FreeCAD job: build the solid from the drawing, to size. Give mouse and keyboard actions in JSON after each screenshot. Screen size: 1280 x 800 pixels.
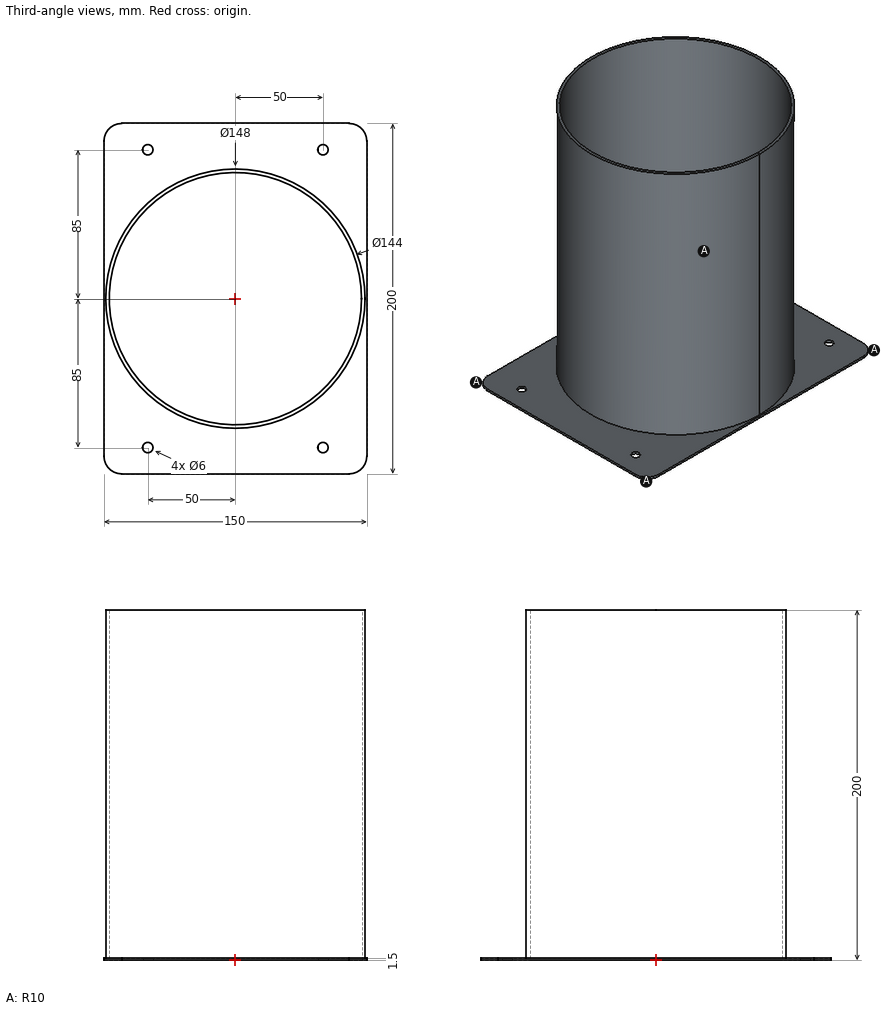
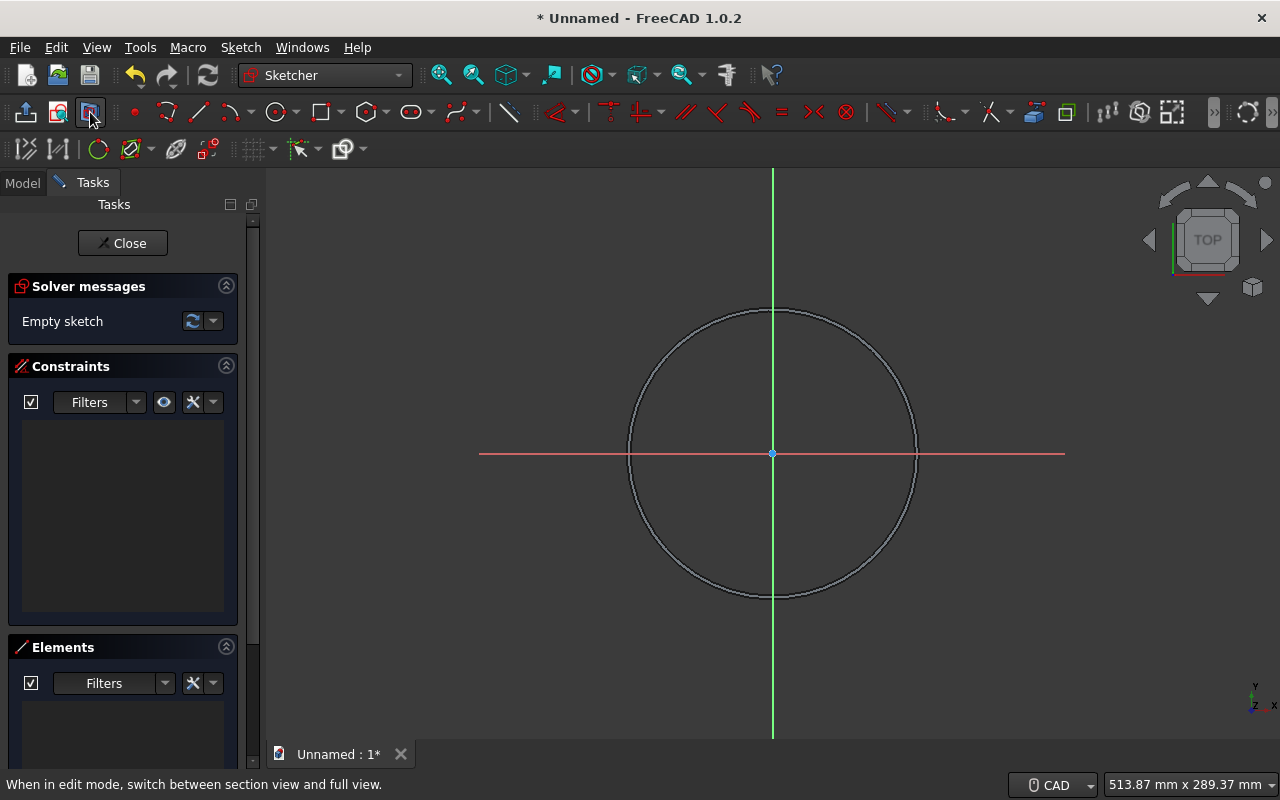
{"action": "left_click", "coordinate": [344, 112]}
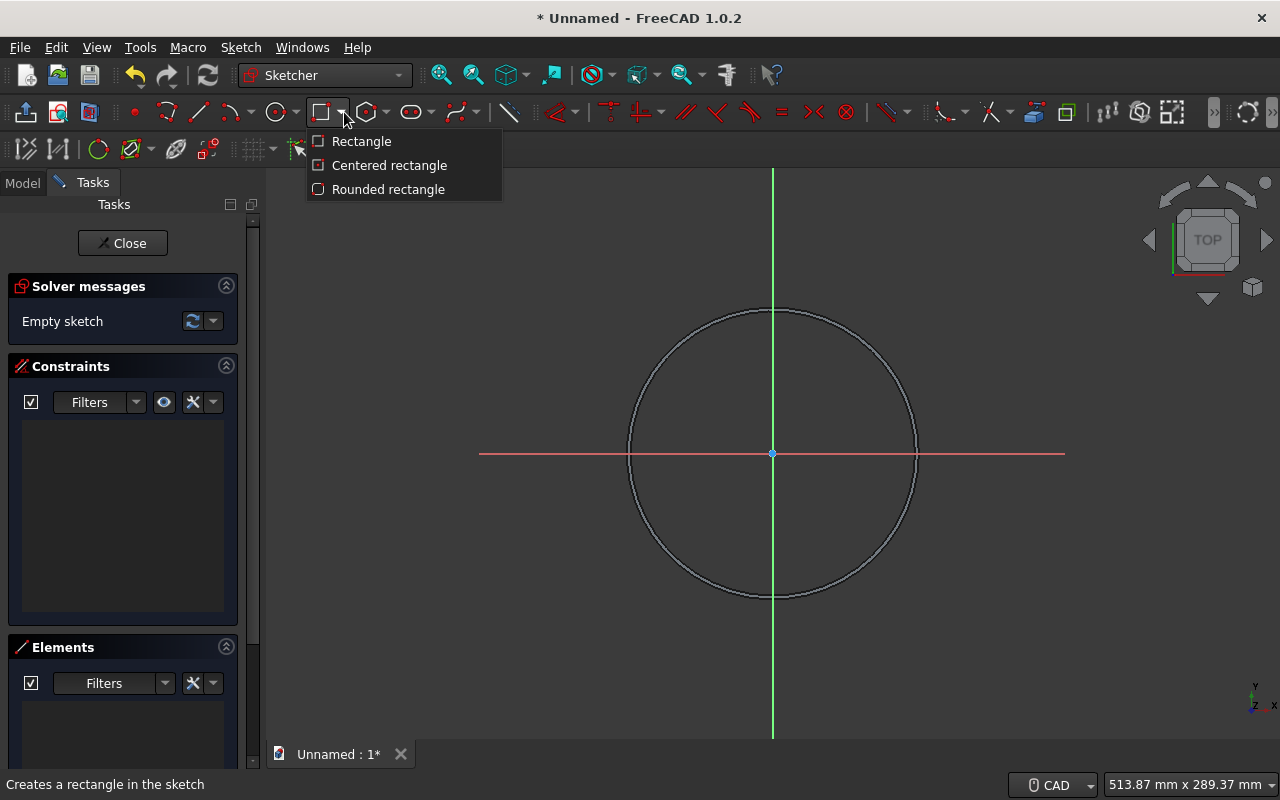
{"action": "left_click", "coordinate": [404, 165]}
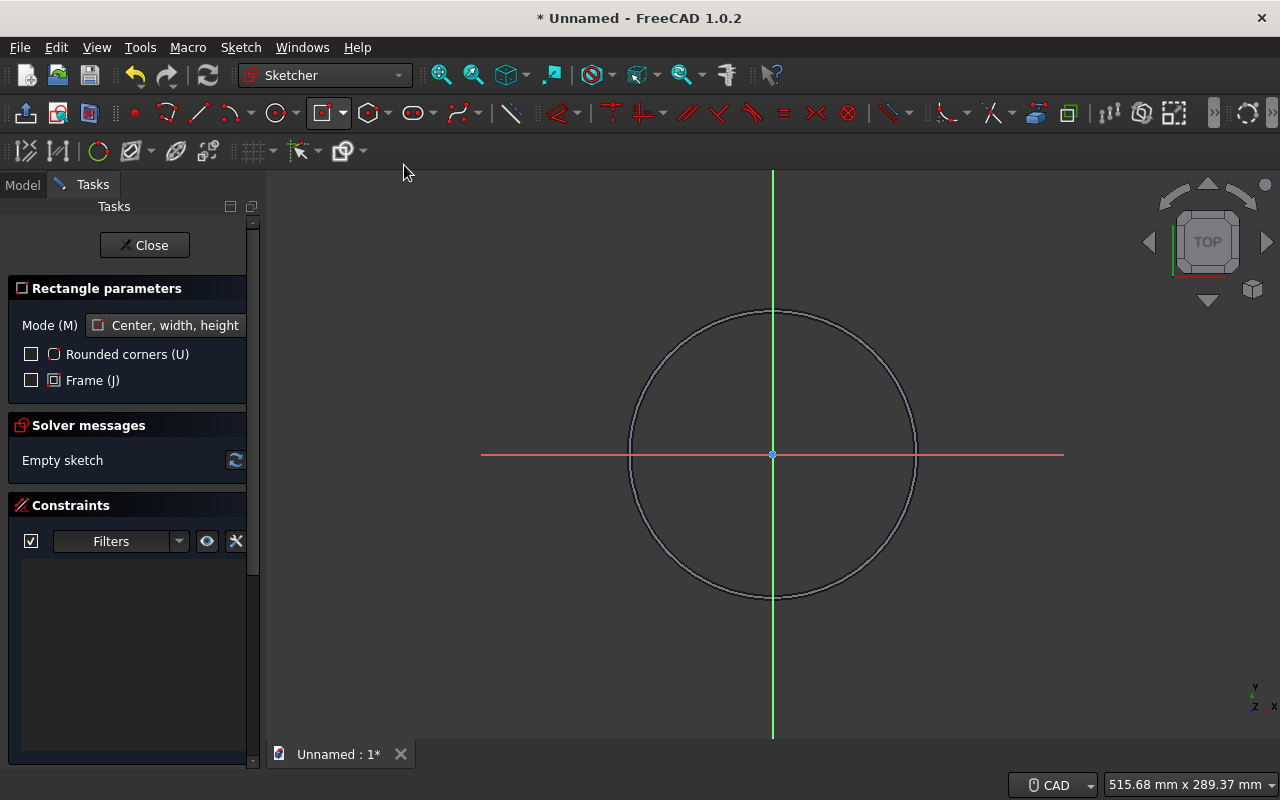
{"action": "left_click", "coordinate": [773, 454]}
{"action": "mouse_move", "coordinate": [920, 258]}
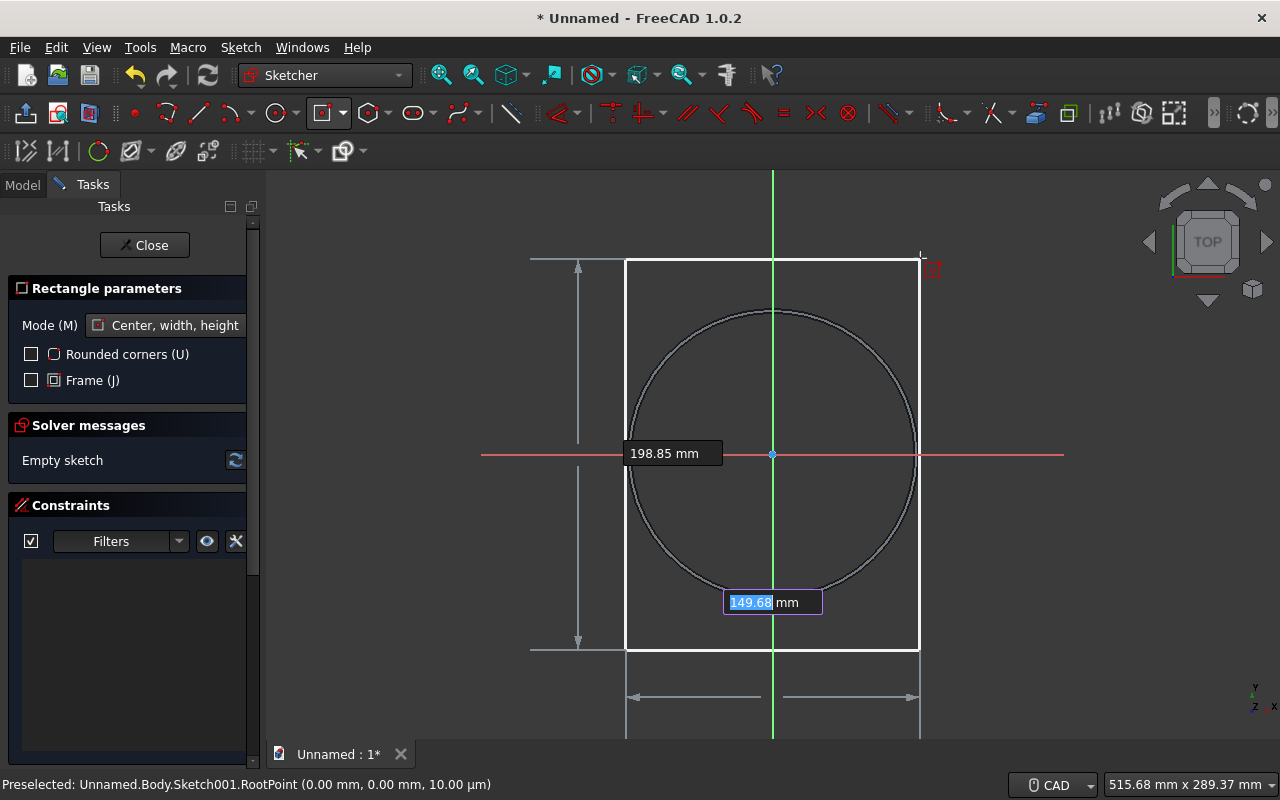
{"action": "type", "text": "150"}
{"action": "key", "text": "Tab"}
{"action": "type", "text": "200"}
{"action": "key", "text": "Return"}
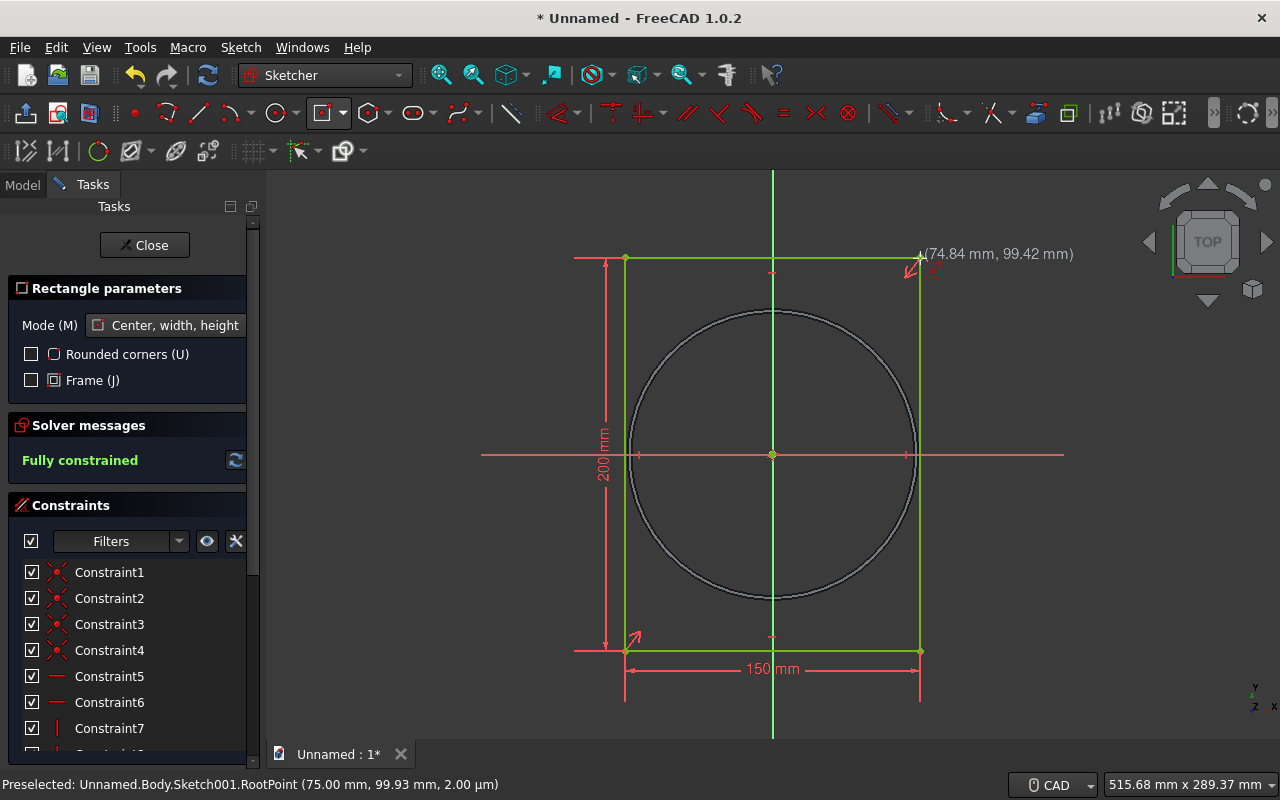
{"action": "left_click", "coordinate": [276, 114]}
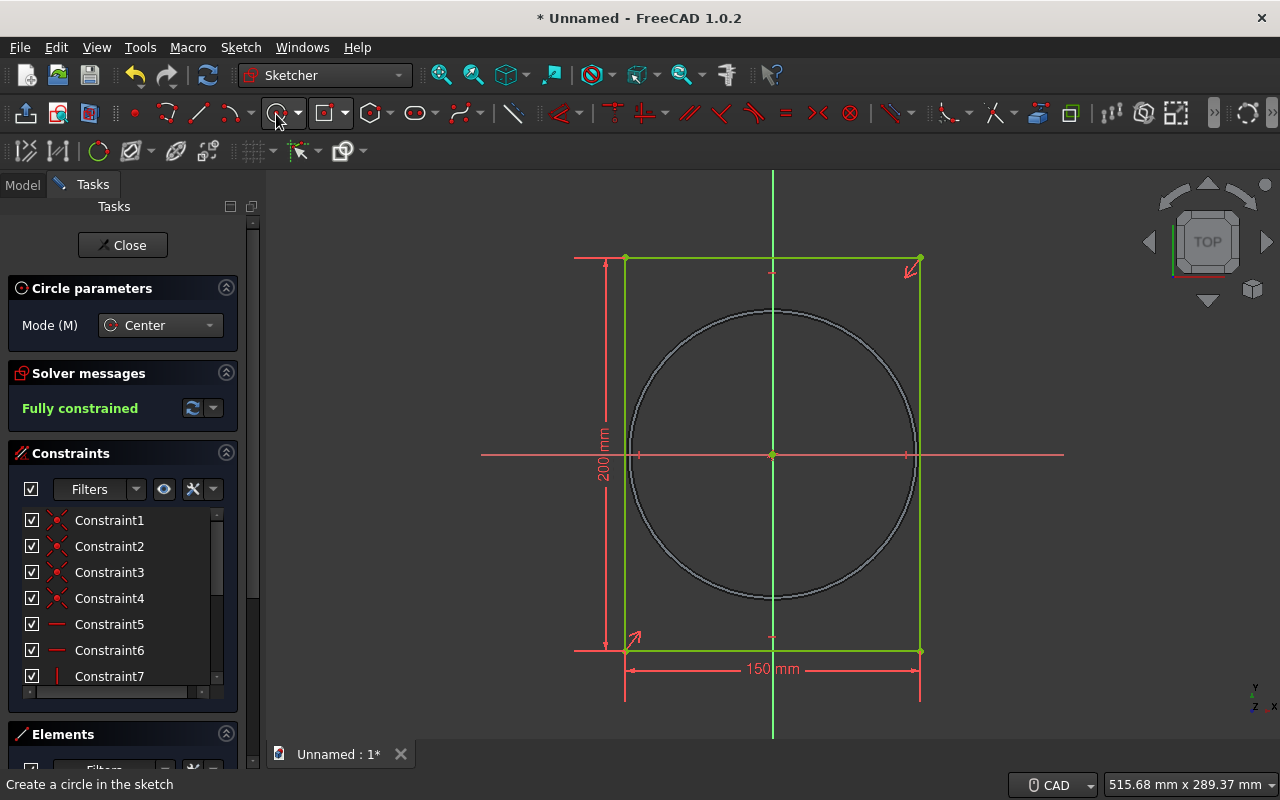
{"action": "left_click", "coordinate": [773, 454]}
{"action": "mouse_move", "coordinate": [876, 352]}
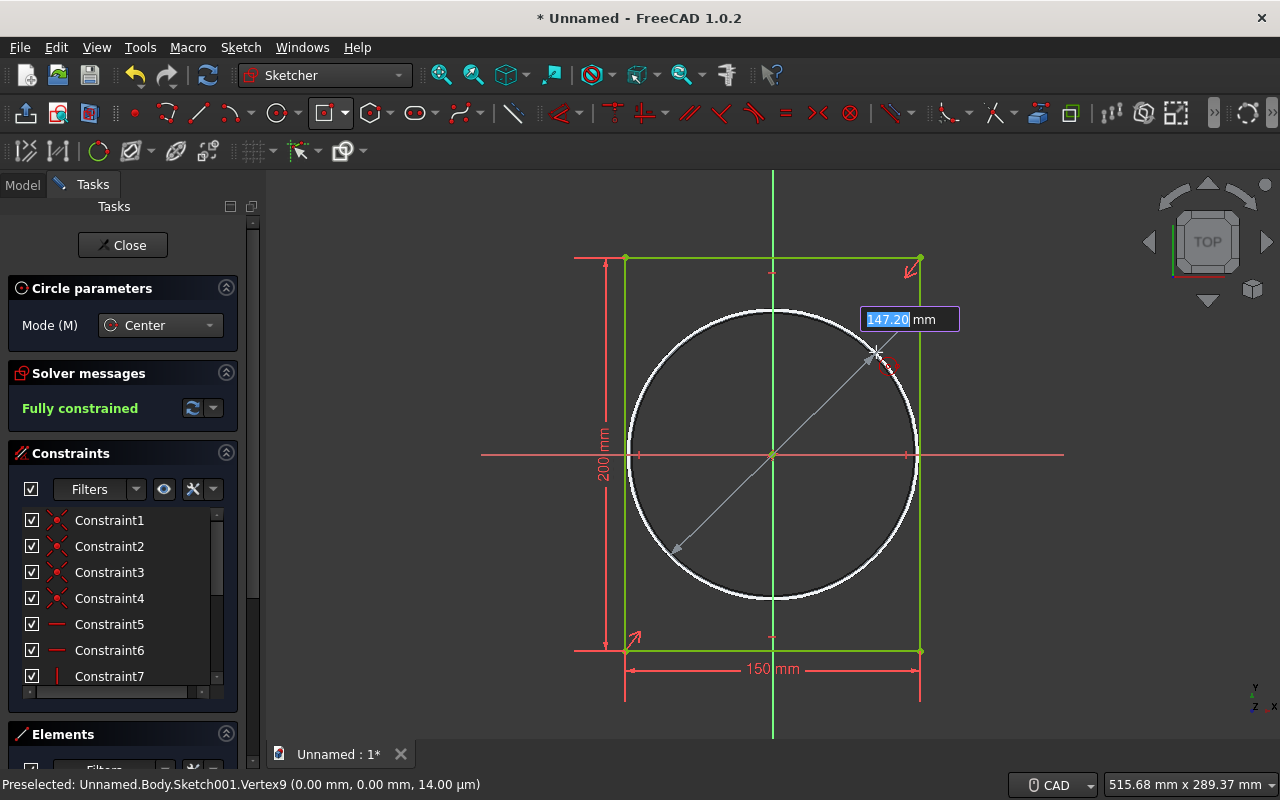
{"action": "type", "text": "148"}
{"action": "key", "text": "Return"}
{"action": "key", "text": "Escape"}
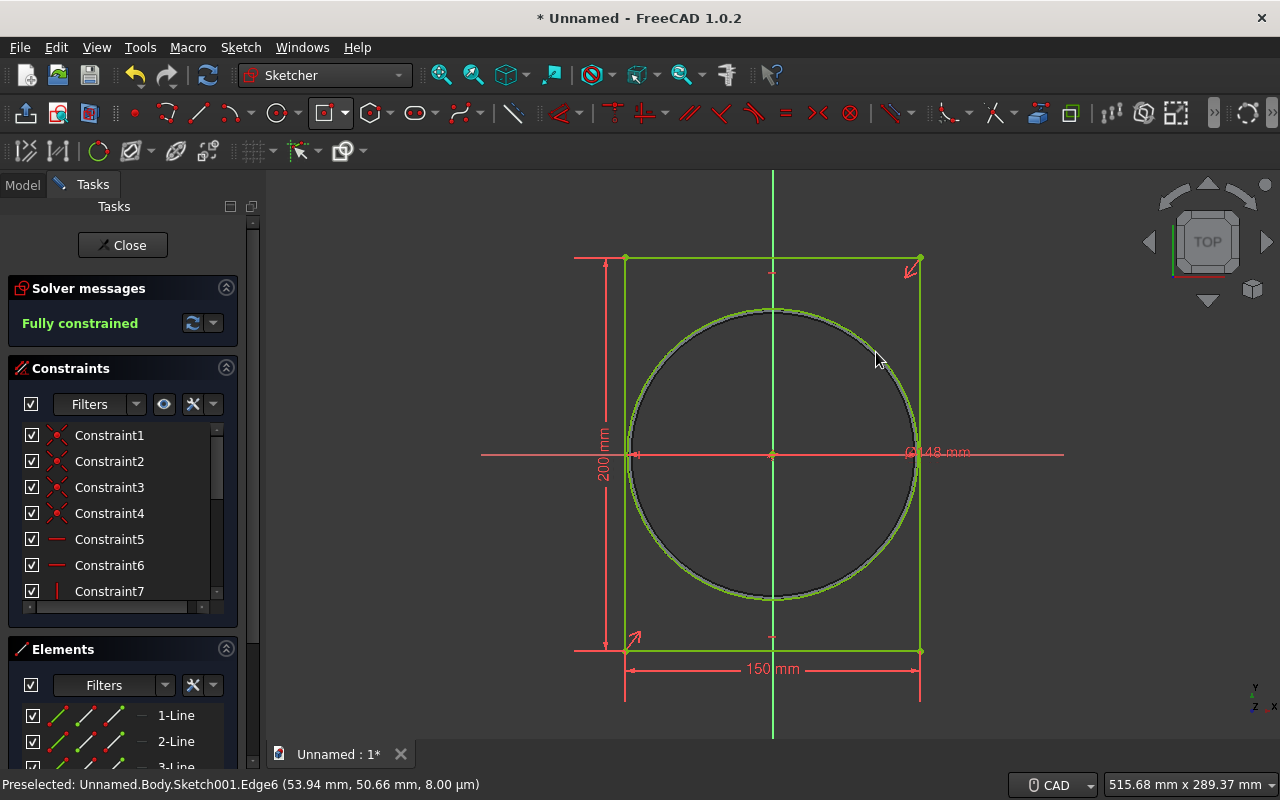
{"action": "left_click", "coordinate": [123, 245]}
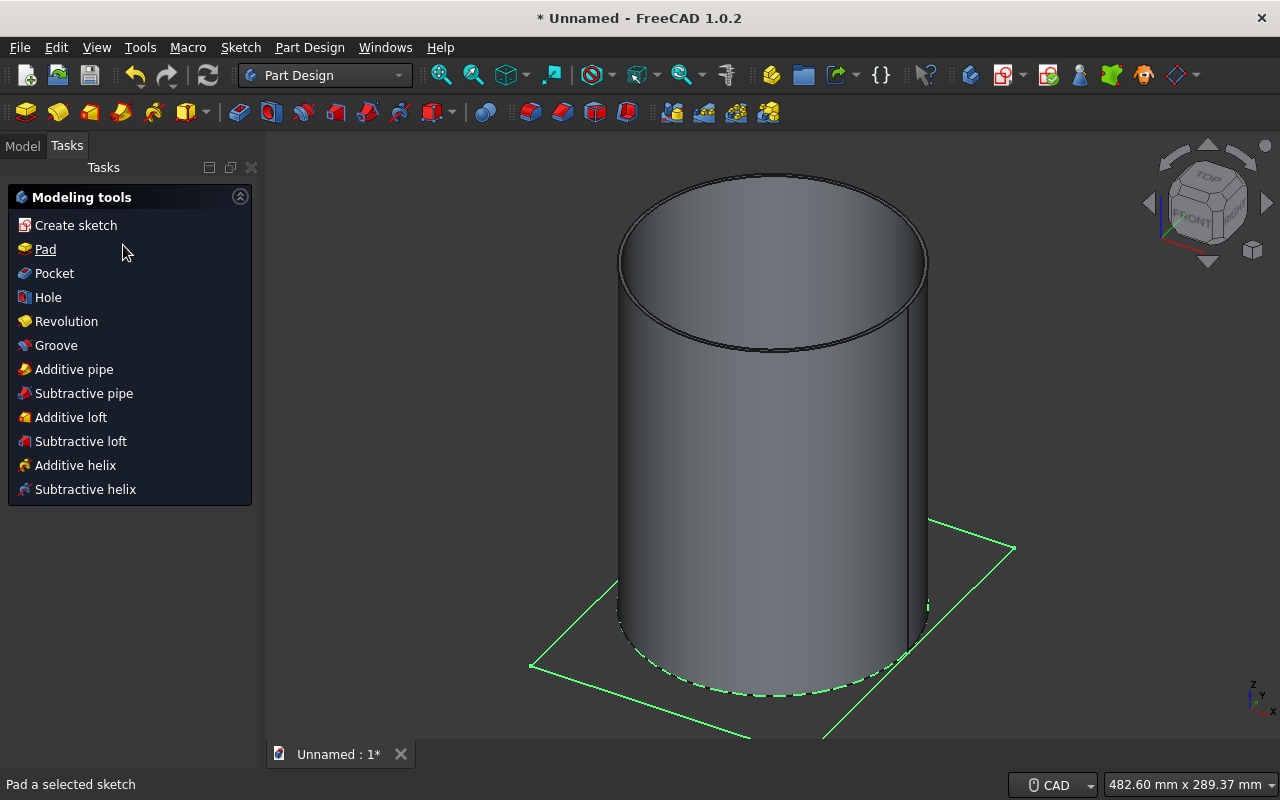
{"action": "left_click", "coordinate": [26, 112]}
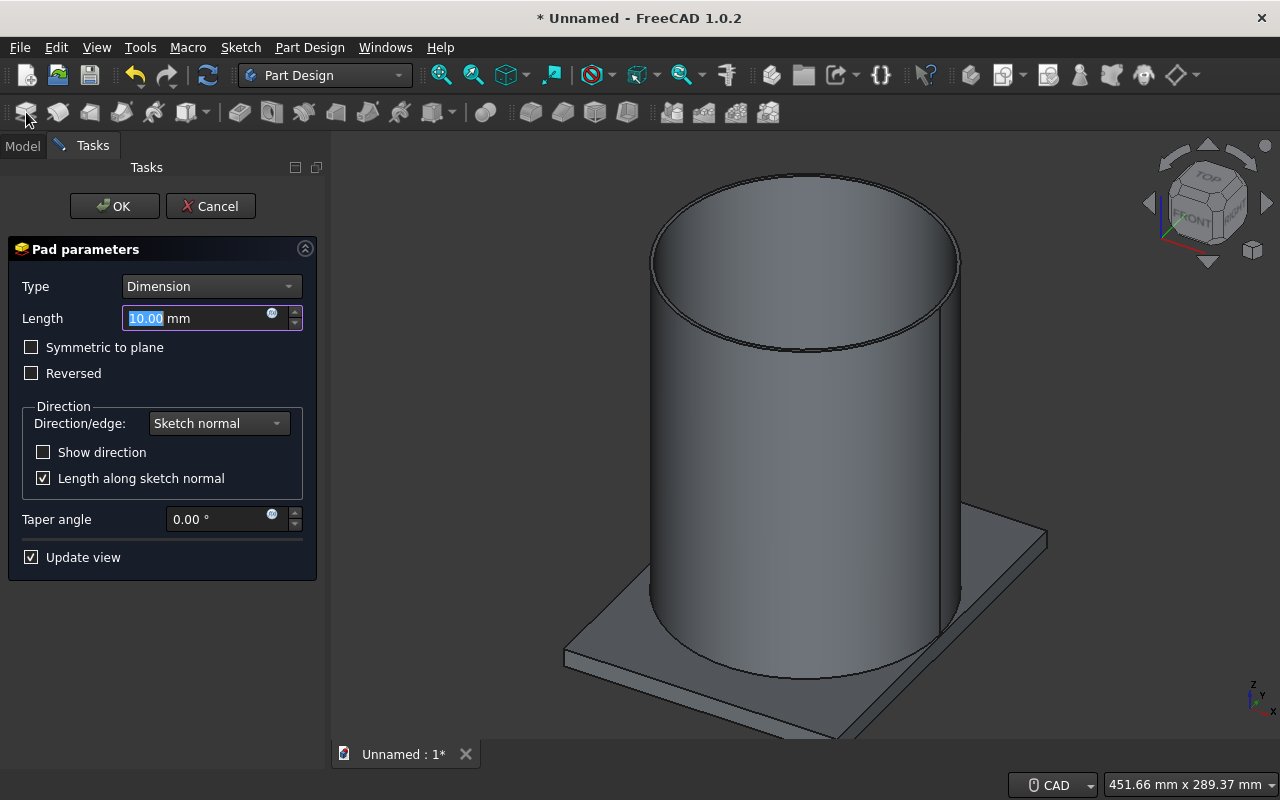
{"action": "type", "text": "1.5"}
{"action": "key", "text": "Tab"}